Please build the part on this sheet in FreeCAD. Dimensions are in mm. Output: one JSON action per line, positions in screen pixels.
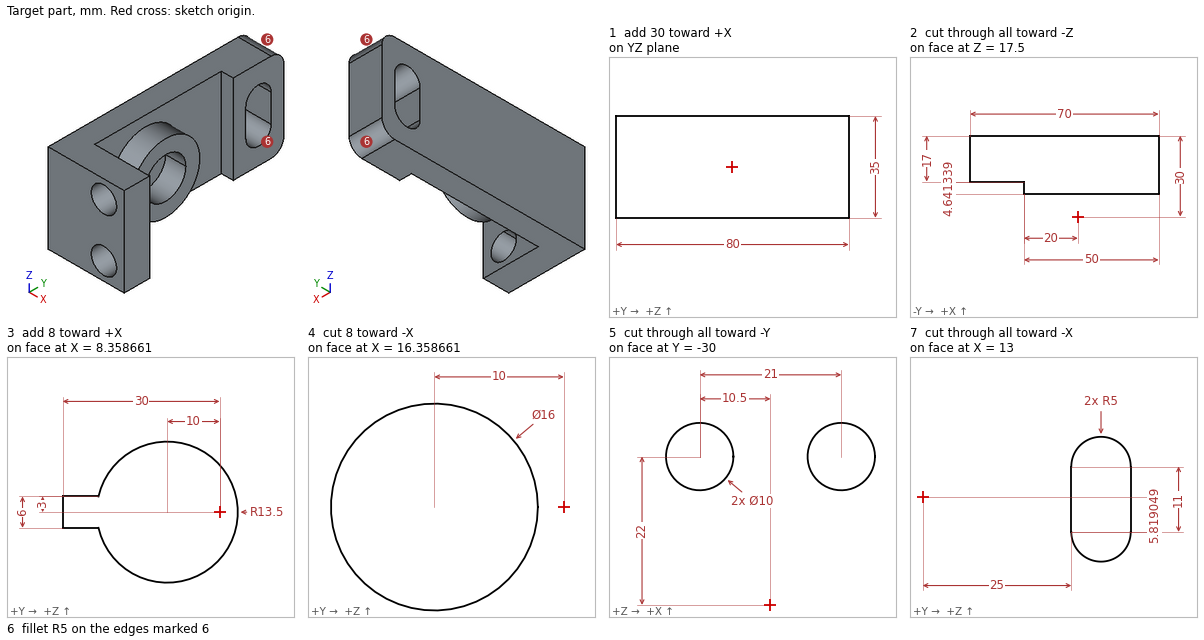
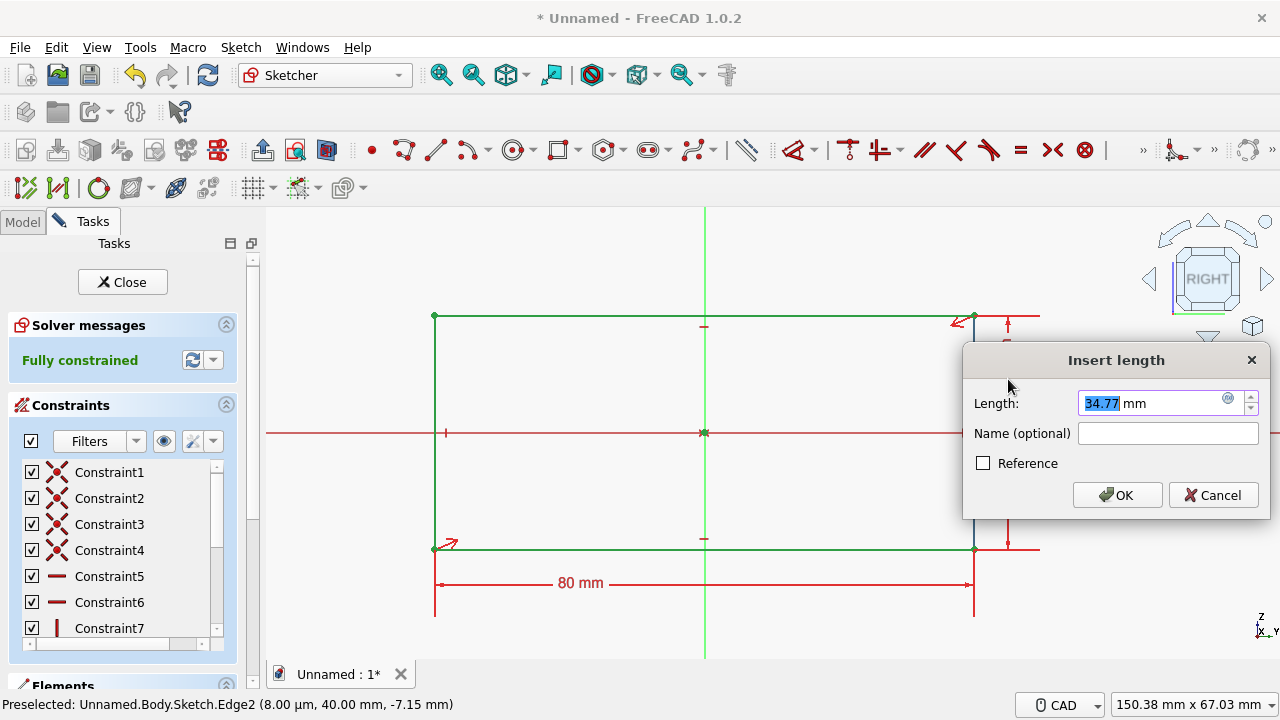
{"action": "type", "text": "35"}
{"action": "key", "text": "Return"}
{"action": "key", "text": "Escape"}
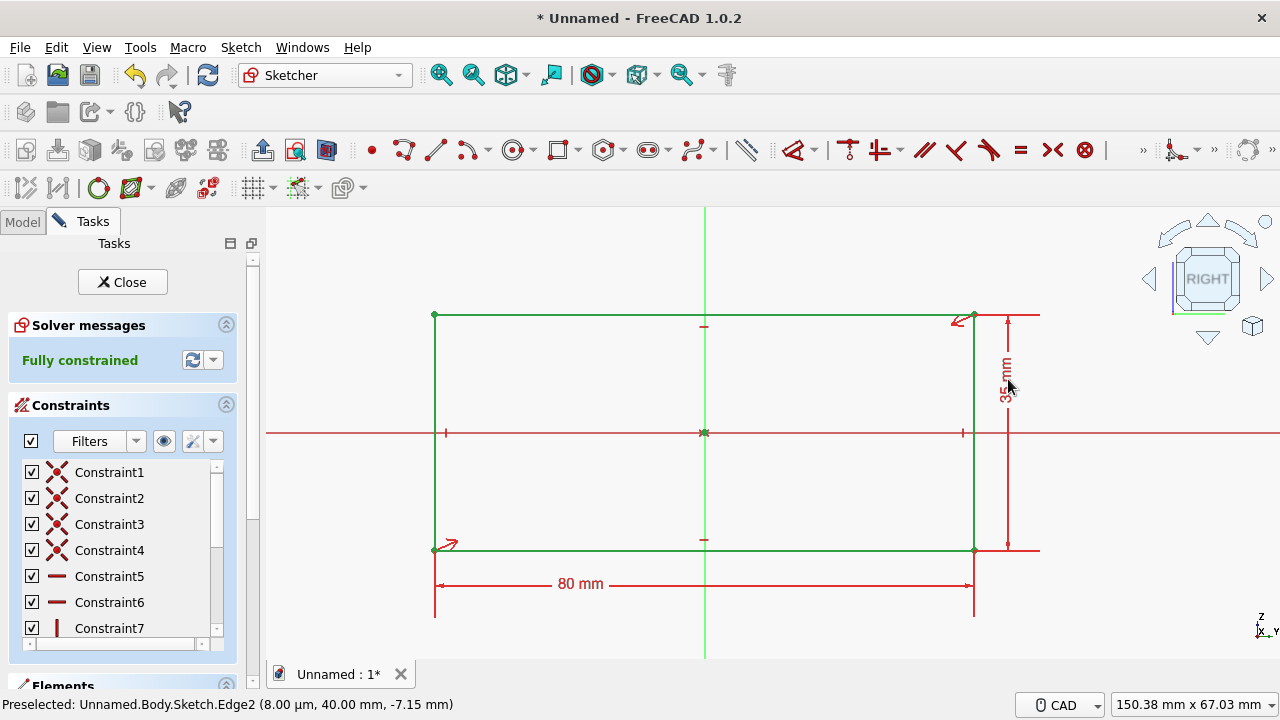
{"action": "left_click", "coordinate": [123, 282]}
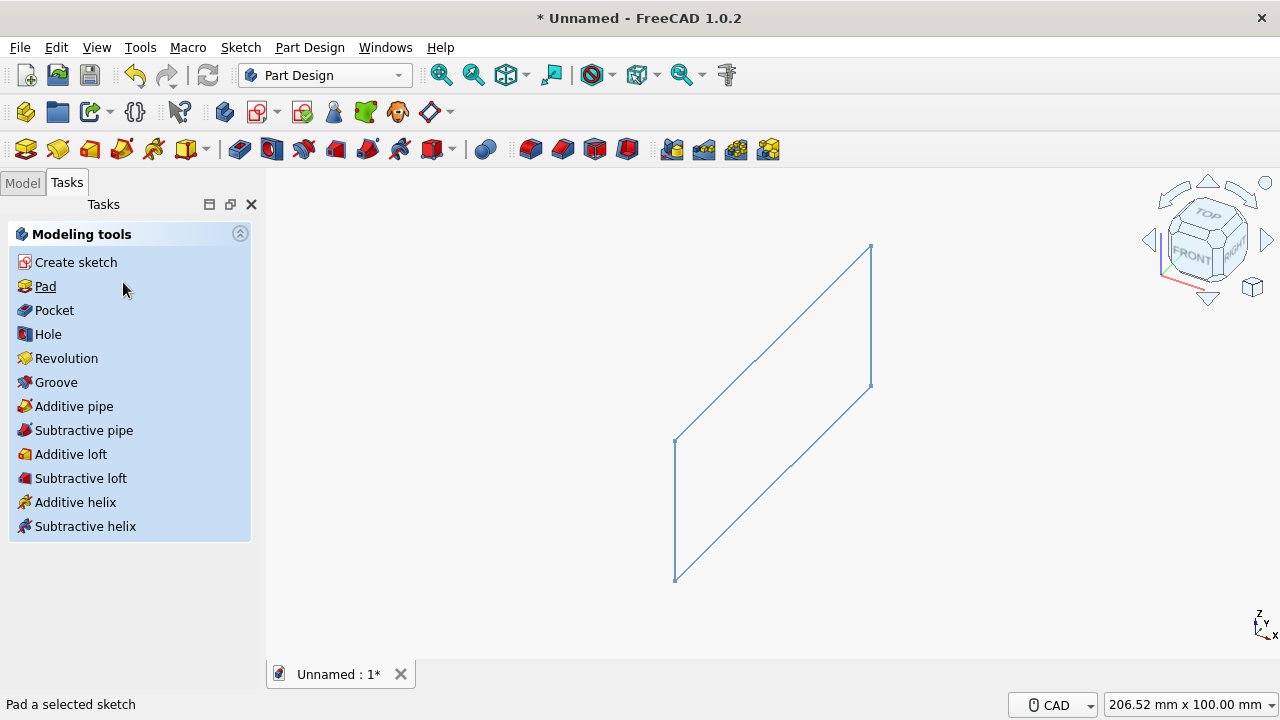
{"action": "left_click", "coordinate": [26, 150]}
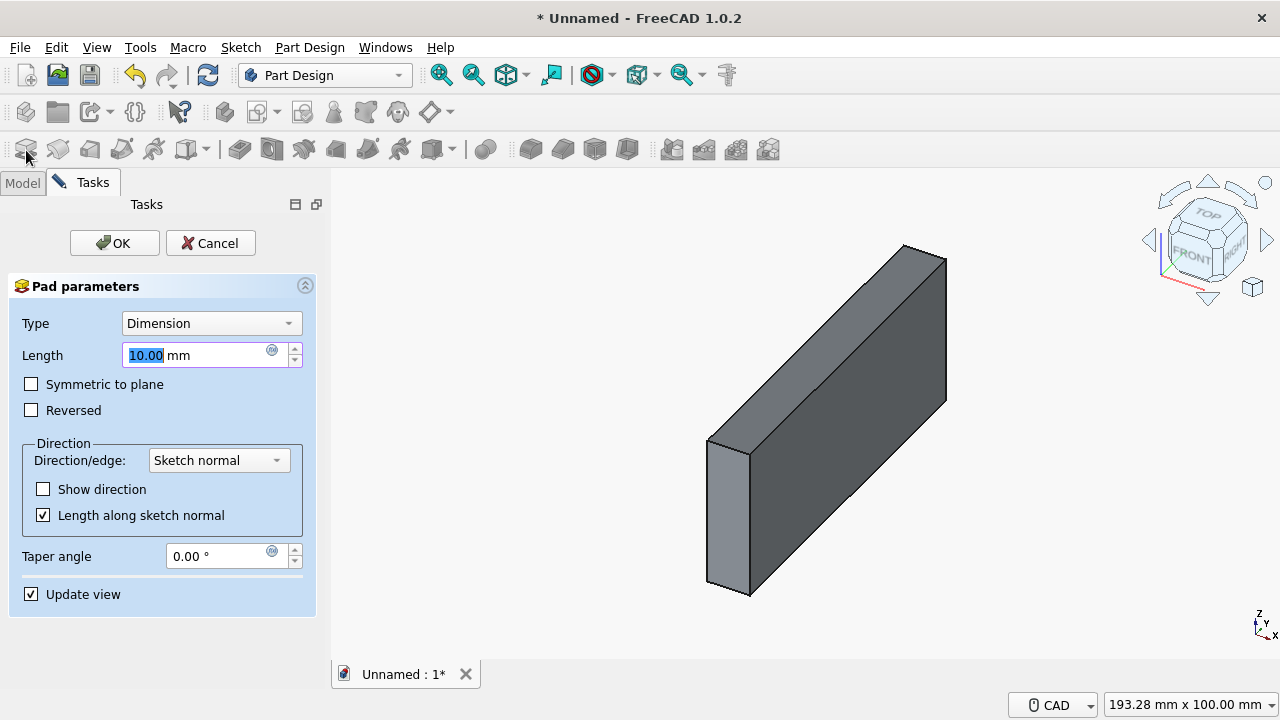
{"action": "type", "text": "30"}
{"action": "key", "text": "Tab"}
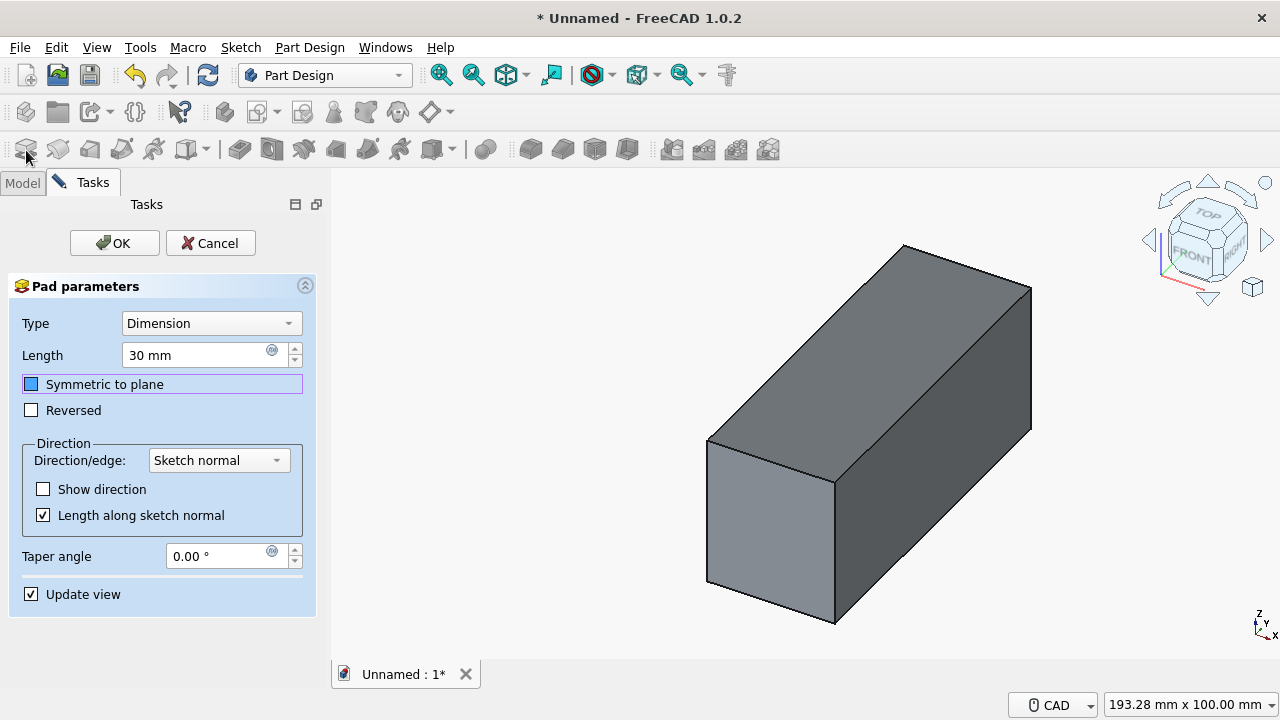
{"action": "left_click", "coordinate": [115, 243]}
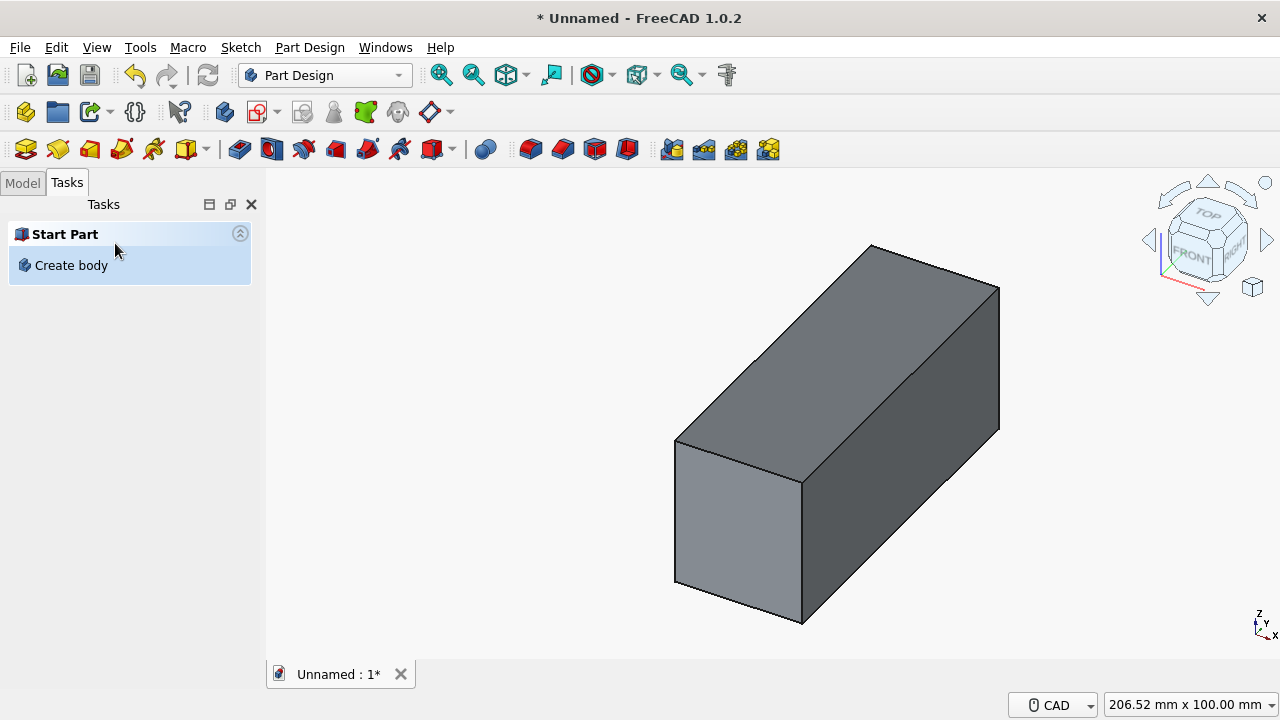
{"action": "left_click", "coordinate": [893, 307]}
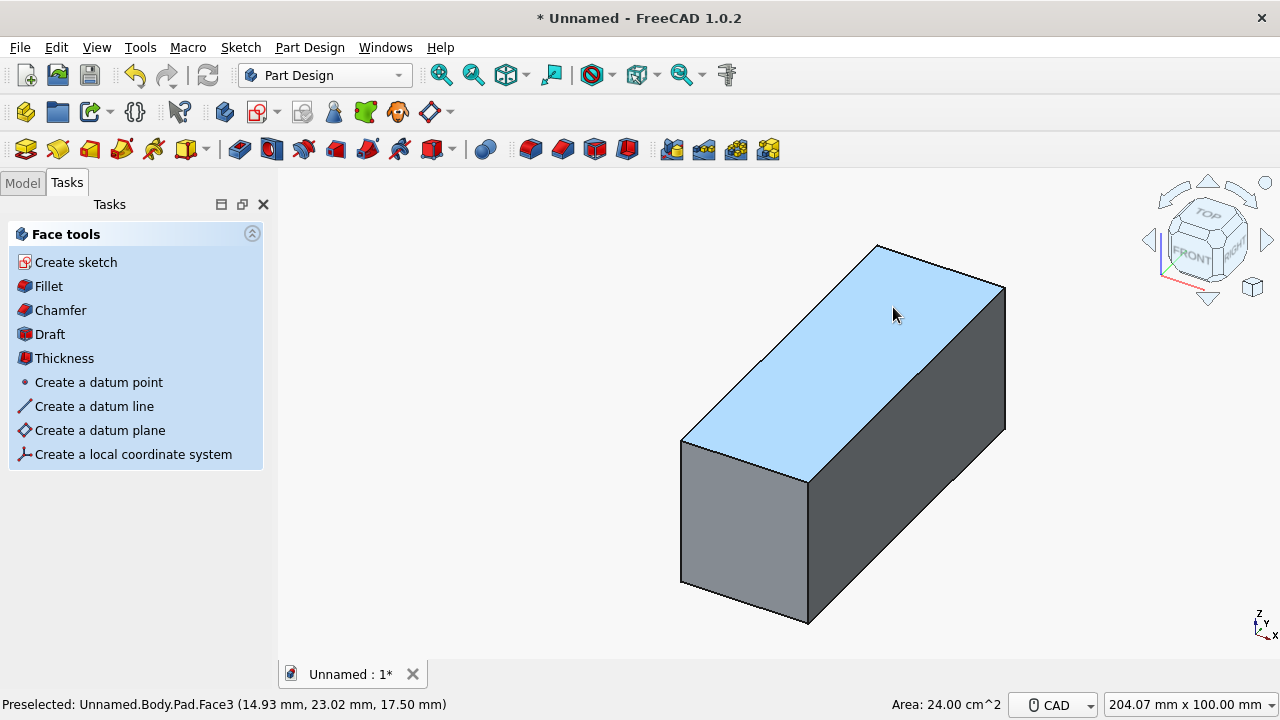
{"action": "left_click", "coordinate": [258, 112]}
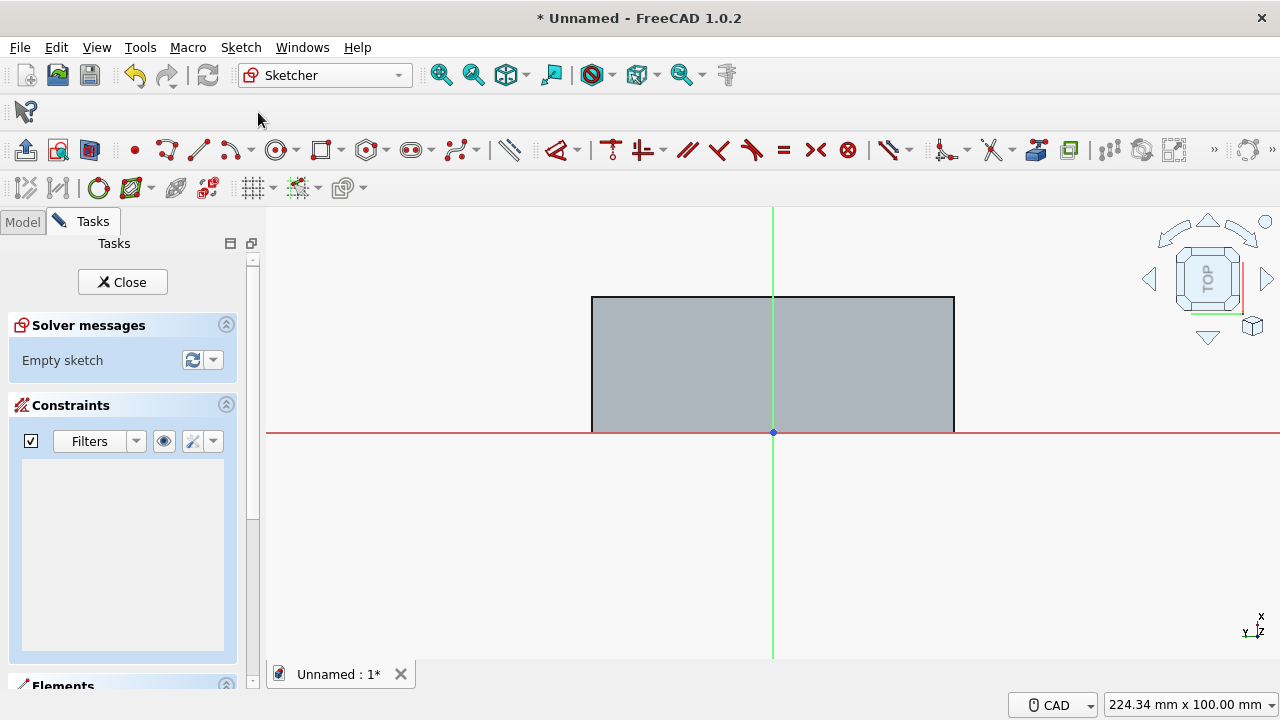
{"action": "scroll", "coordinate": [806, 283], "scroll_direction": "up", "scroll_amount": 3}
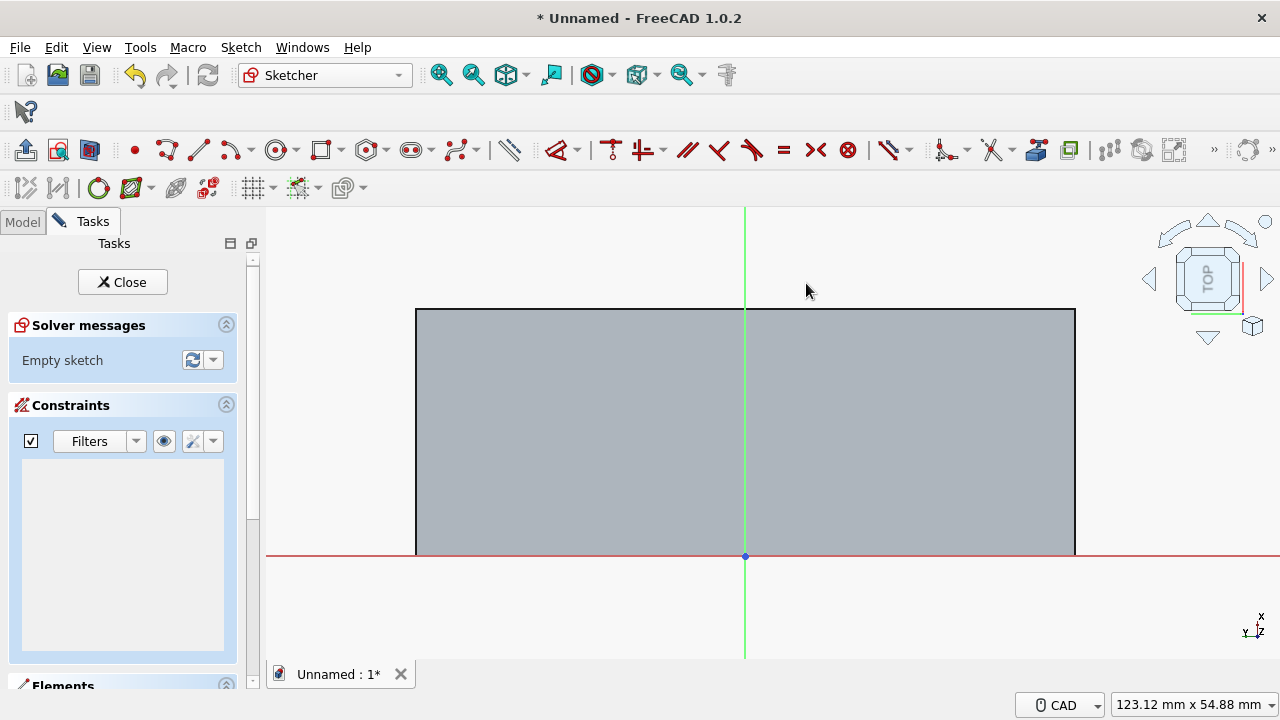
{"action": "left_click", "coordinate": [168, 150]}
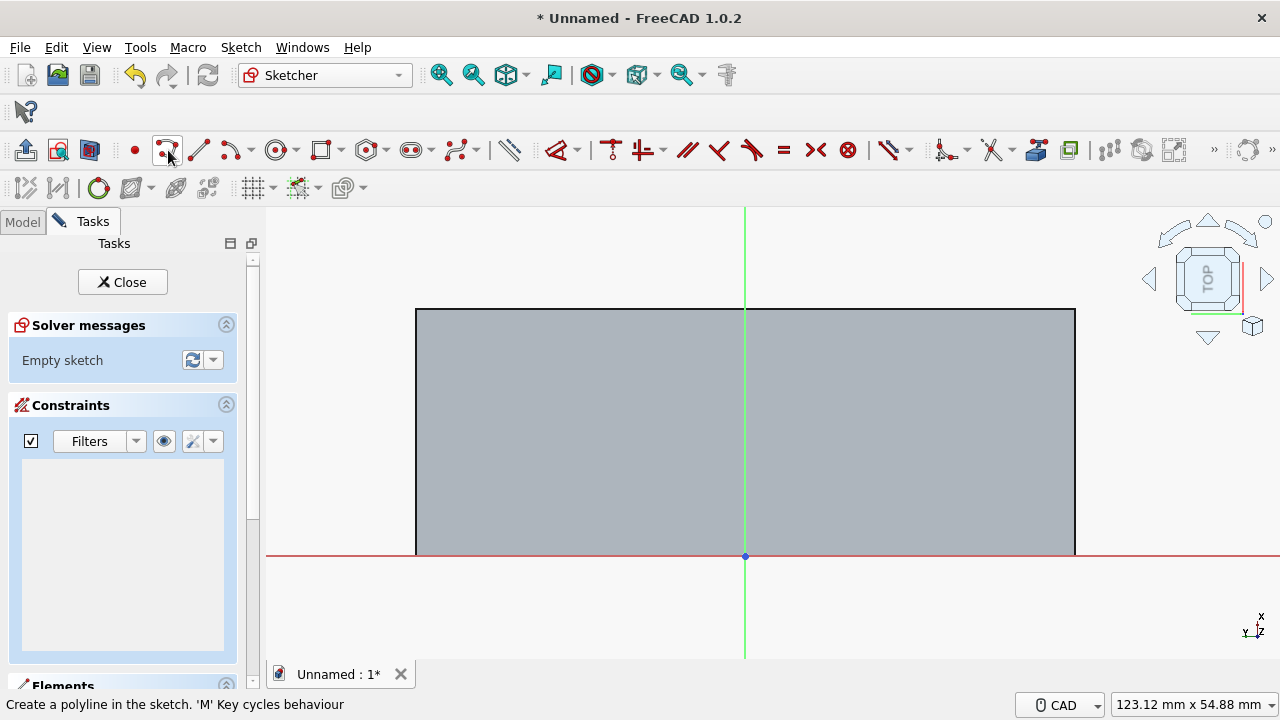
{"action": "left_click", "coordinate": [581, 487]}
{"action": "left_click", "coordinate": [993, 487]}
{"action": "left_click", "coordinate": [993, 309]}
{"action": "left_click", "coordinate": [416, 309]}
{"action": "left_click", "coordinate": [416, 449]}
{"action": "left_click", "coordinate": [581, 449]}
{"action": "left_click", "coordinate": [581, 488]}
{"action": "key", "text": "Escape"}
{"action": "key", "text": "Escape"}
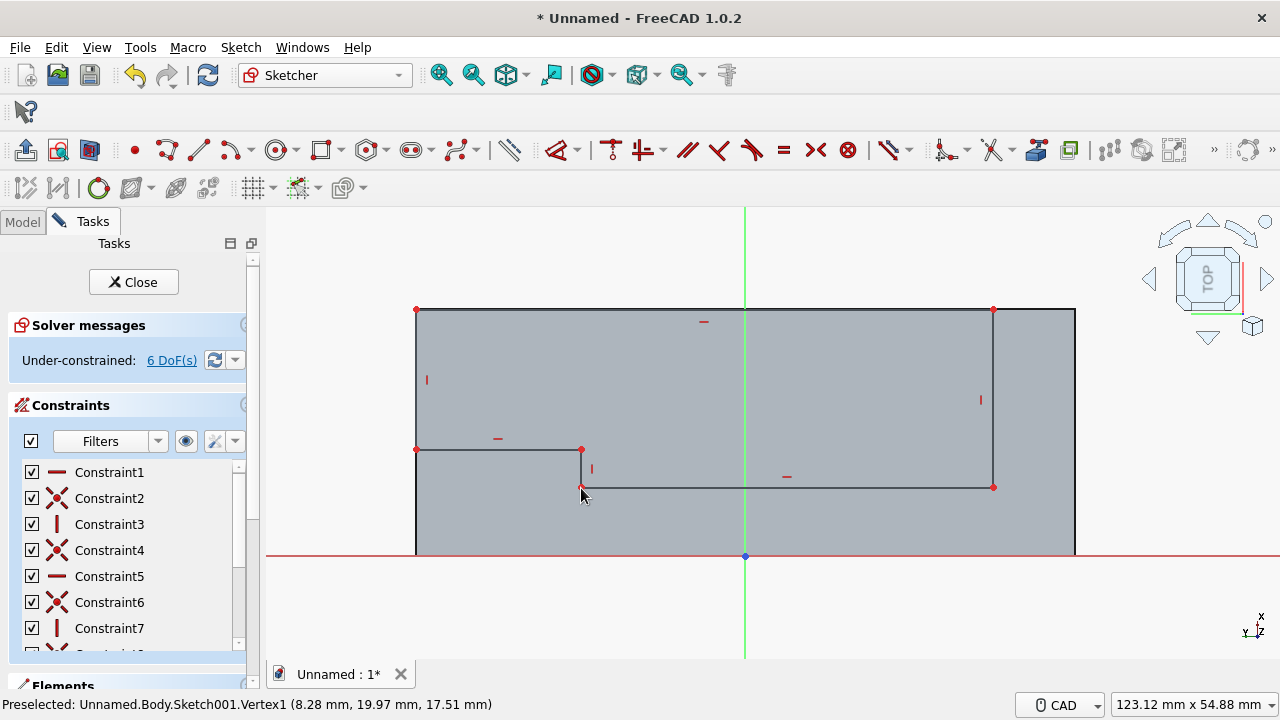
{"action": "left_click", "coordinate": [556, 150]}